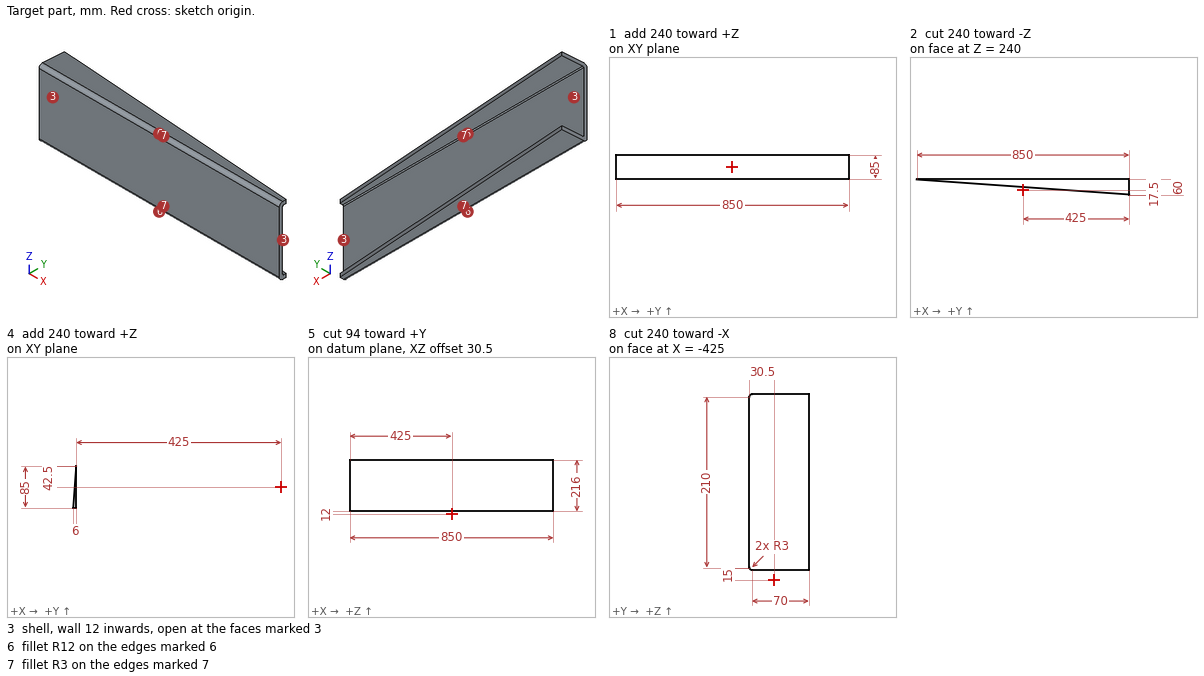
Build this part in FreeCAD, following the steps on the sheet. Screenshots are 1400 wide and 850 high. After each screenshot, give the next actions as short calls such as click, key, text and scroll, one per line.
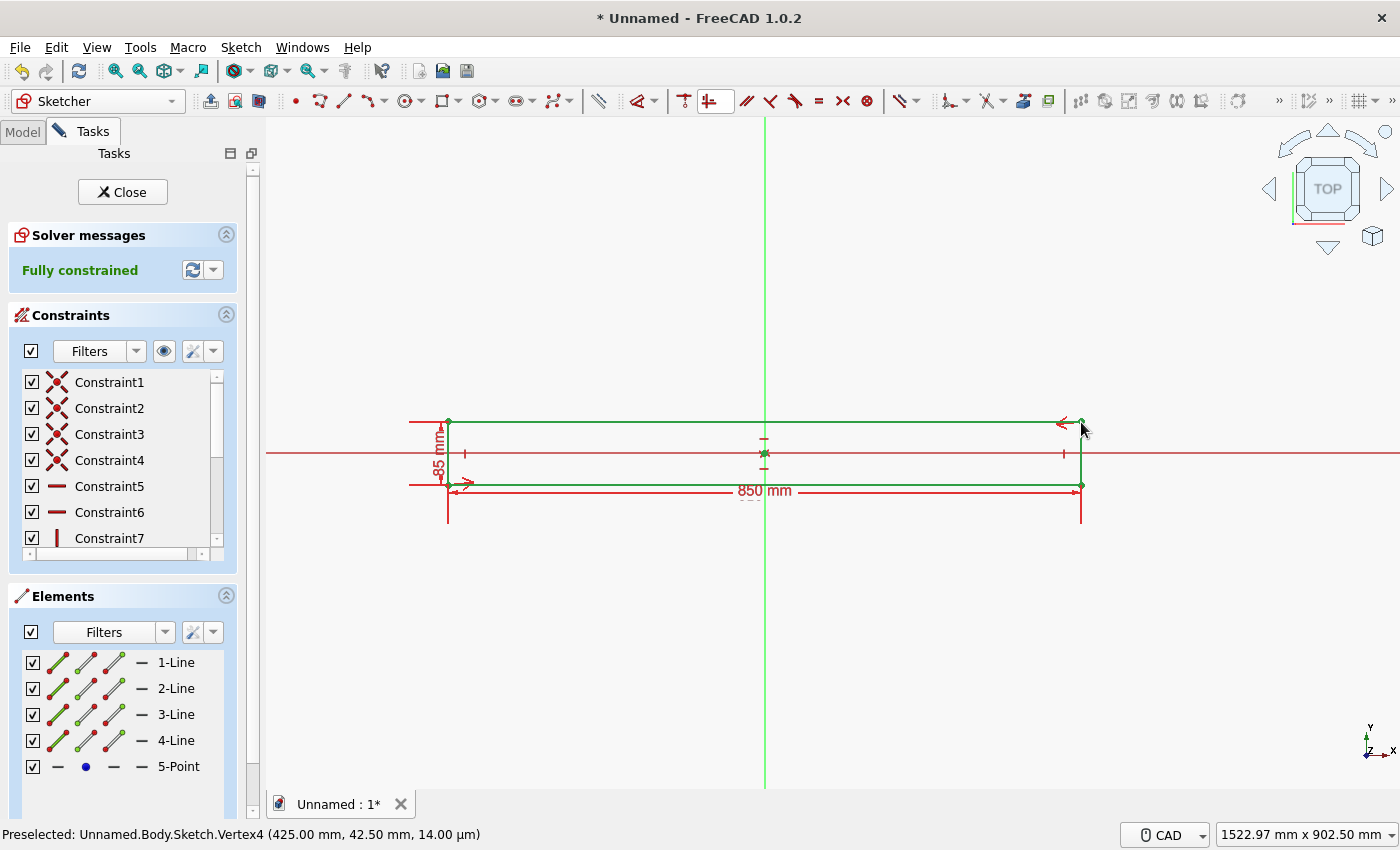
click(123, 192)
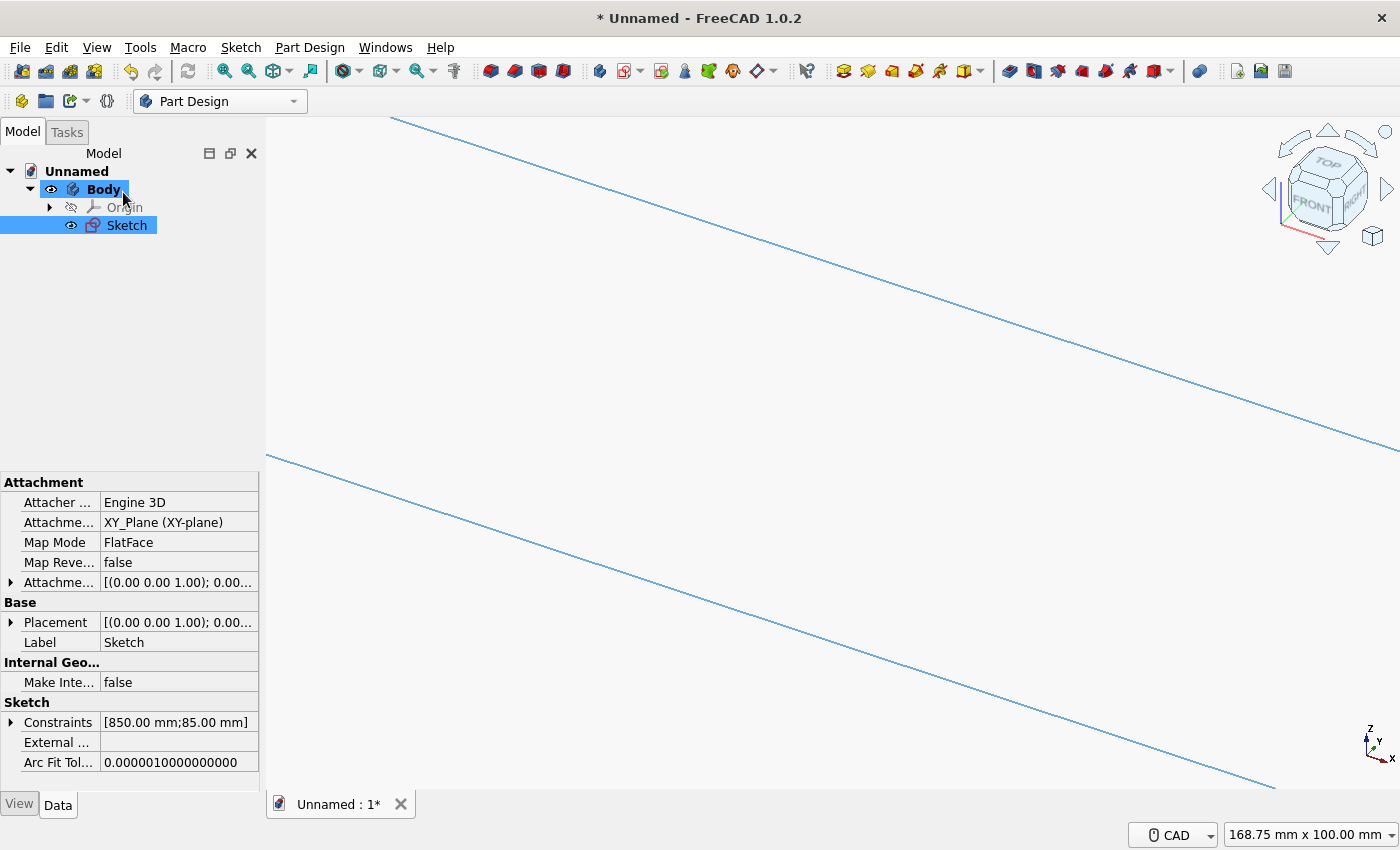
click(844, 72)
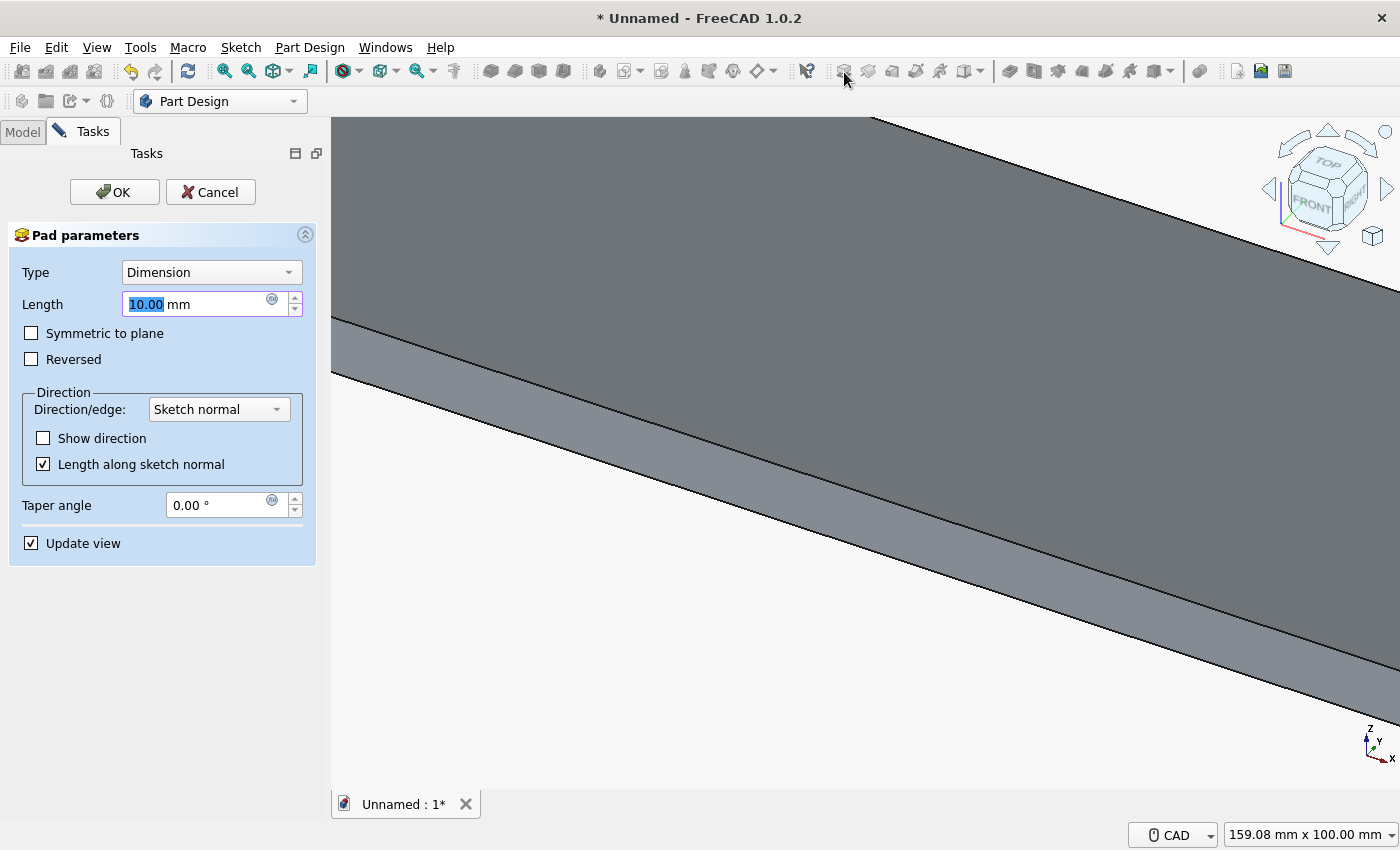
text(240)
key(Tab)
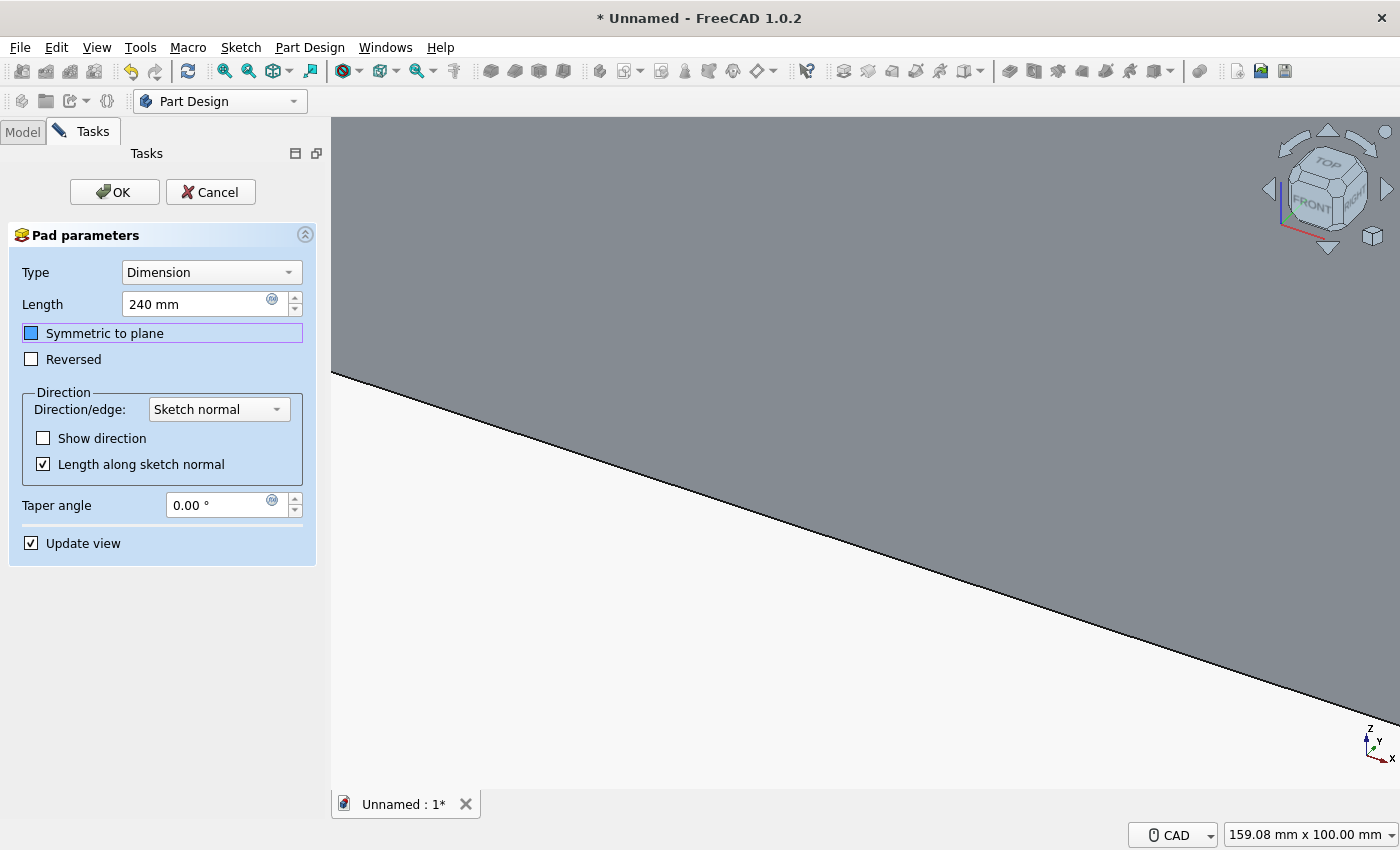
click(115, 192)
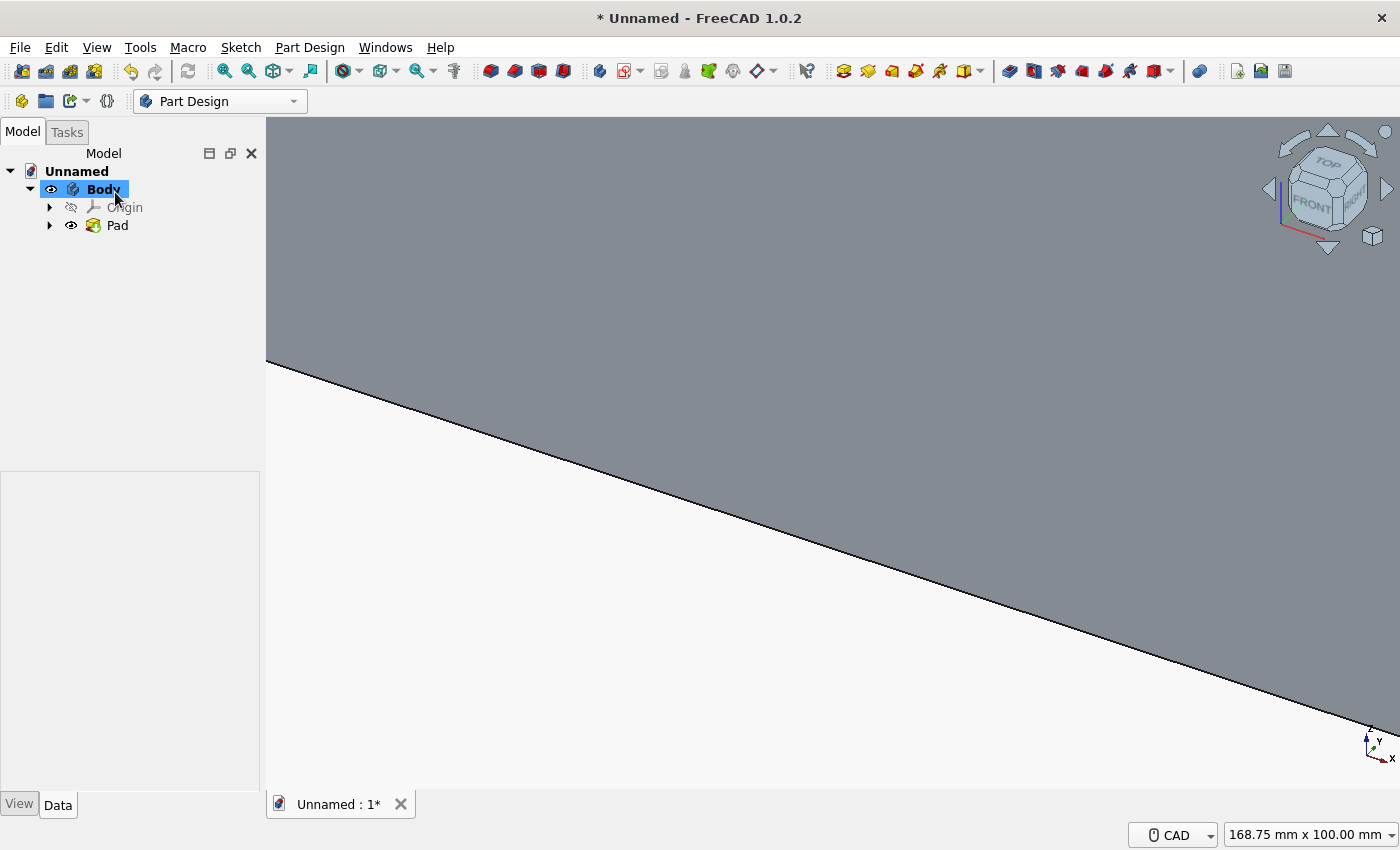
key(v)
key(f)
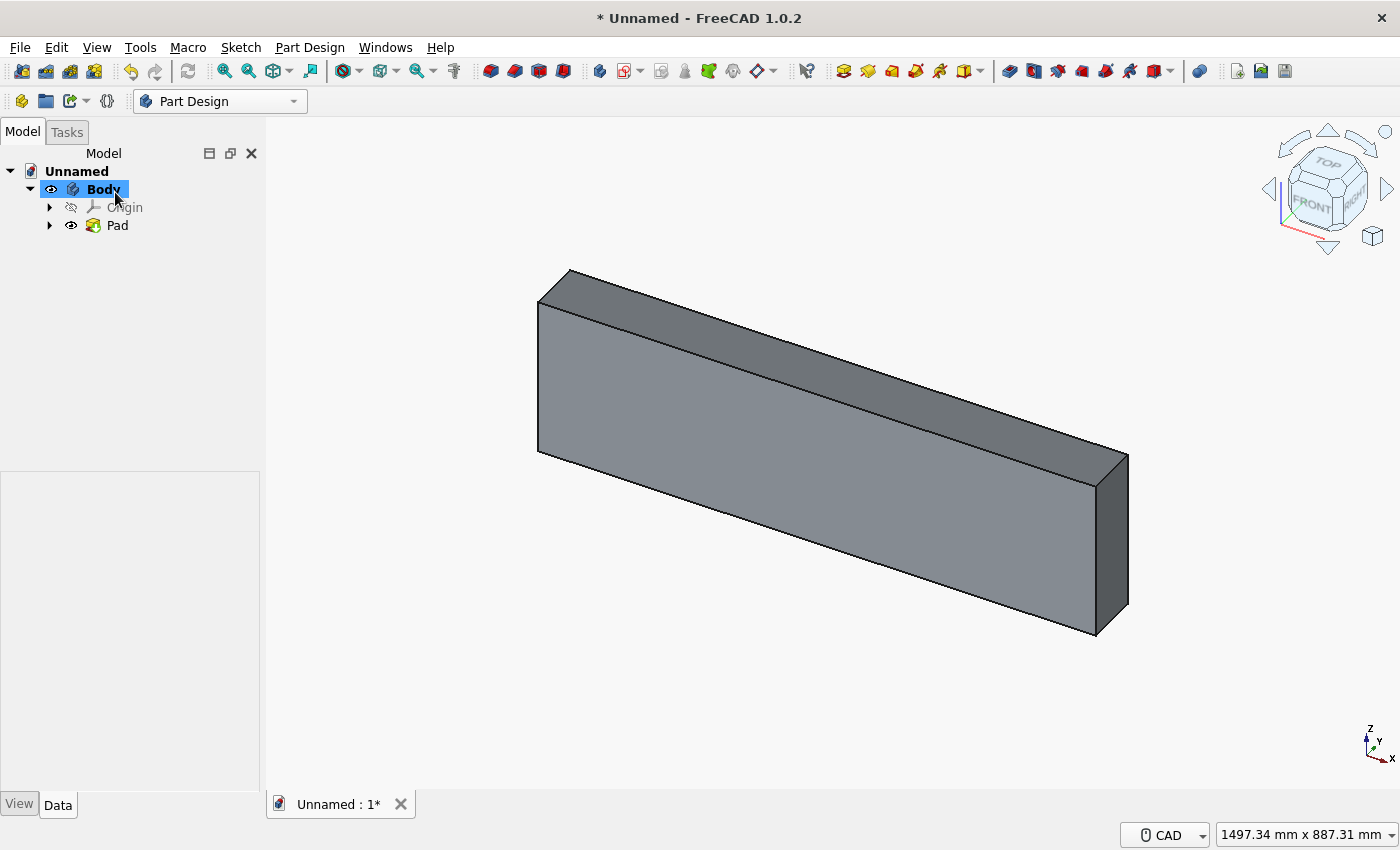
click(1072, 457)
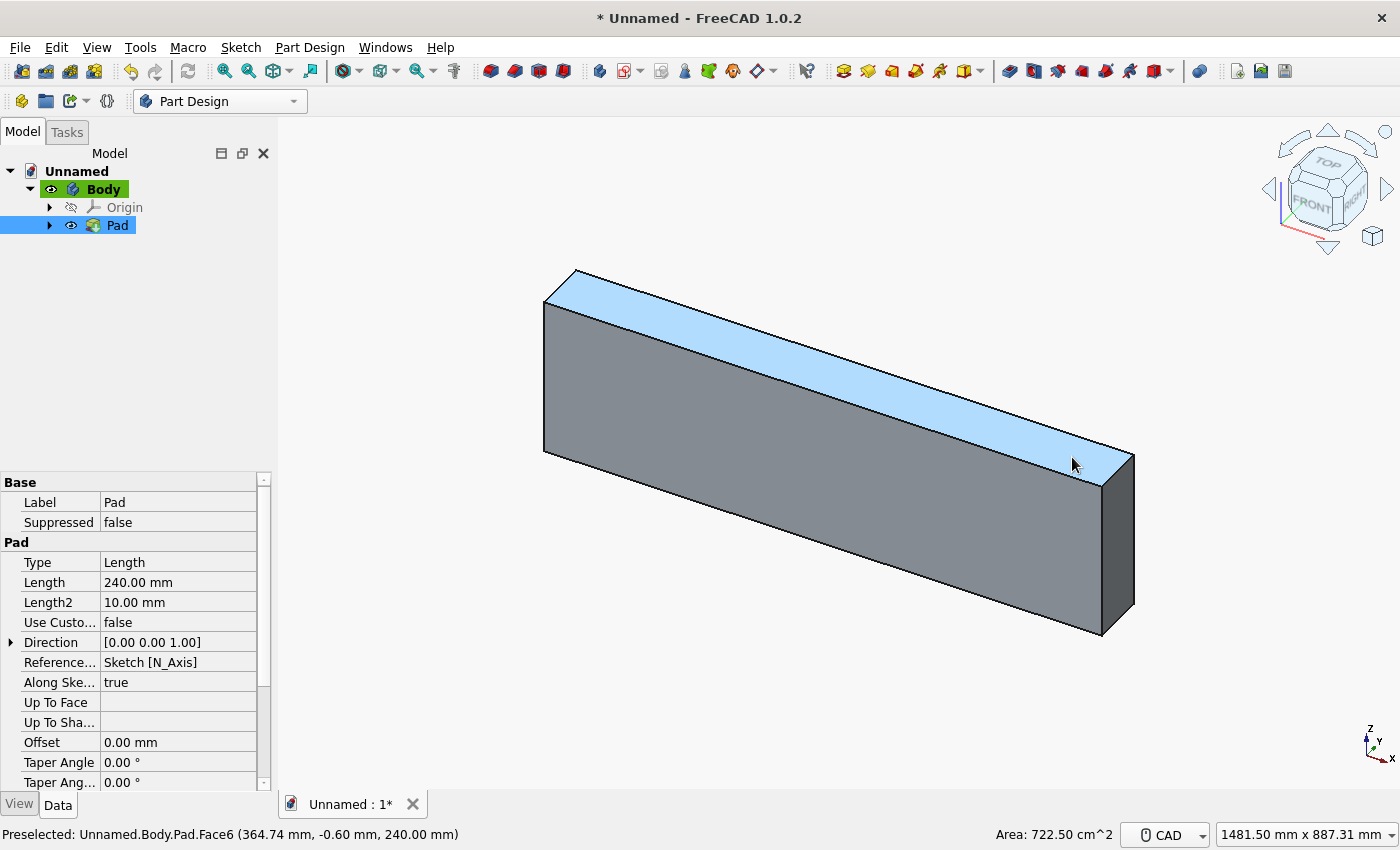
click(624, 72)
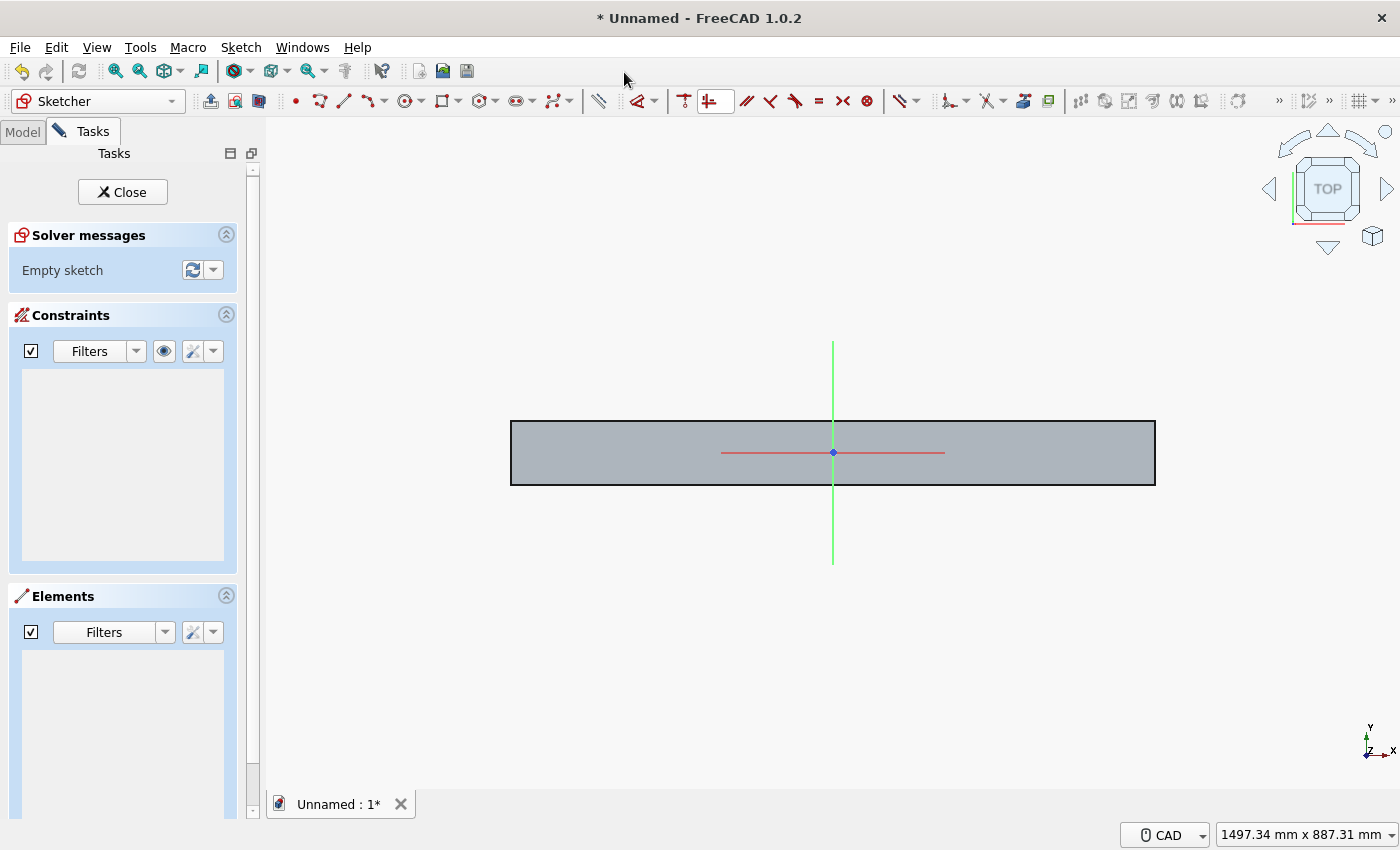
key(g)
key(m)